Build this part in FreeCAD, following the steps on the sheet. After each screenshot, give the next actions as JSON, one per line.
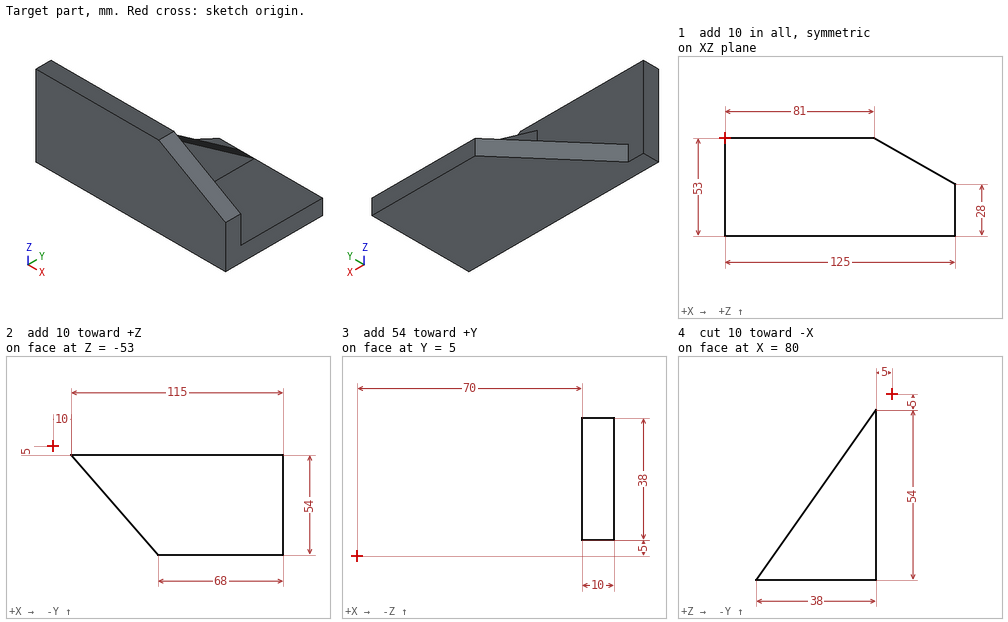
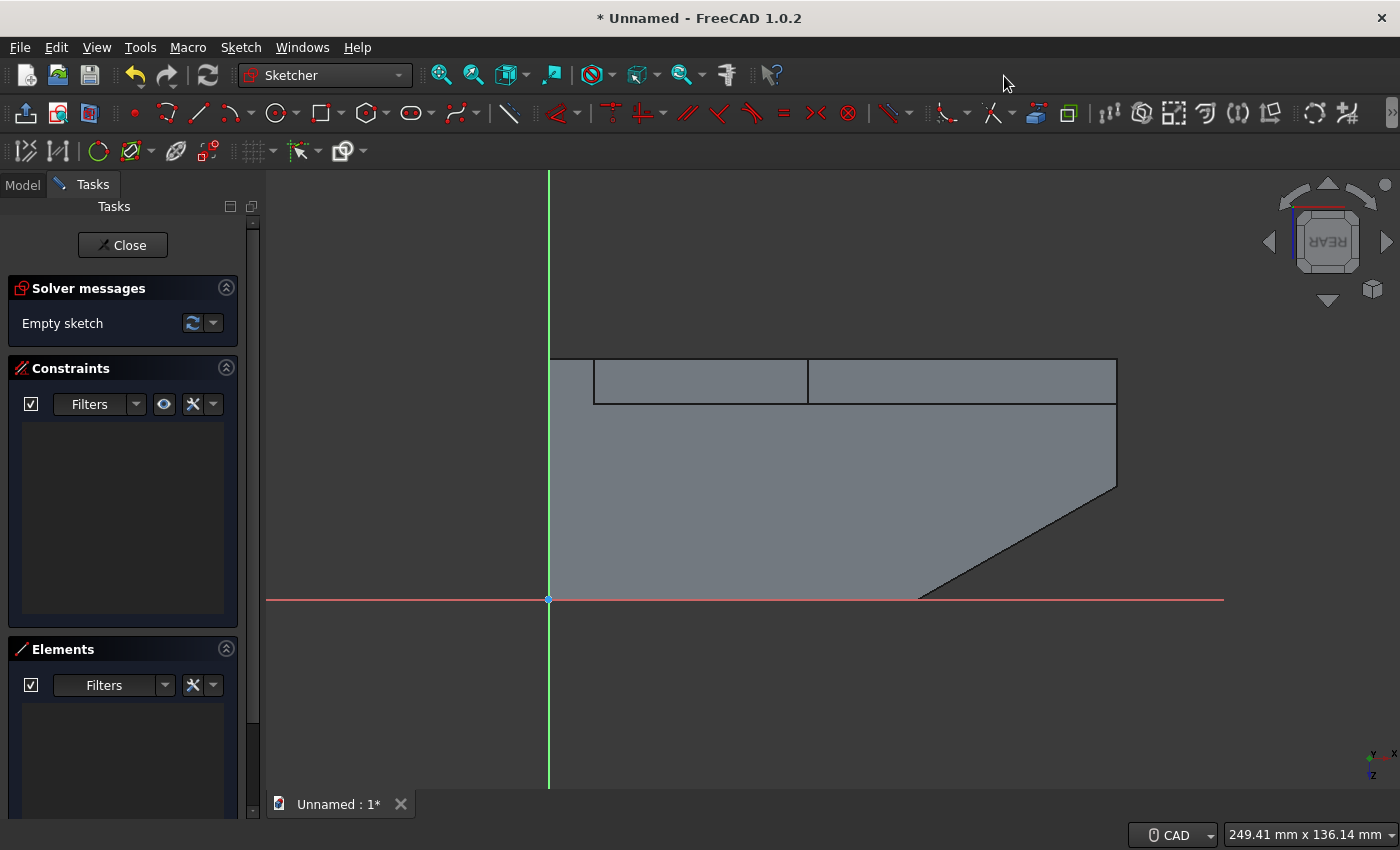
{"action": "scroll", "coordinate": [690, 530], "scroll_direction": "up", "scroll_amount": 3}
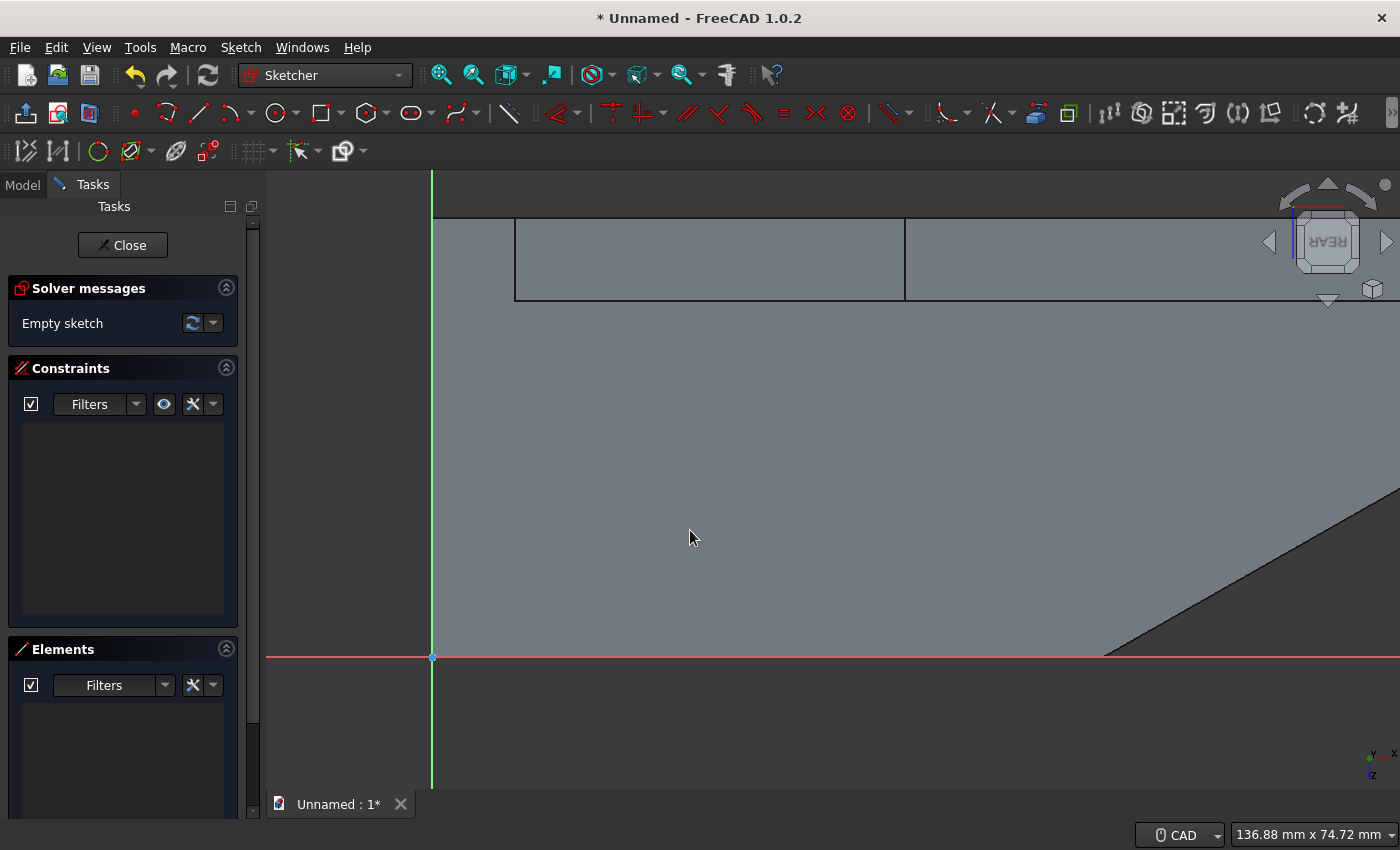
{"action": "left_click", "coordinate": [322, 114]}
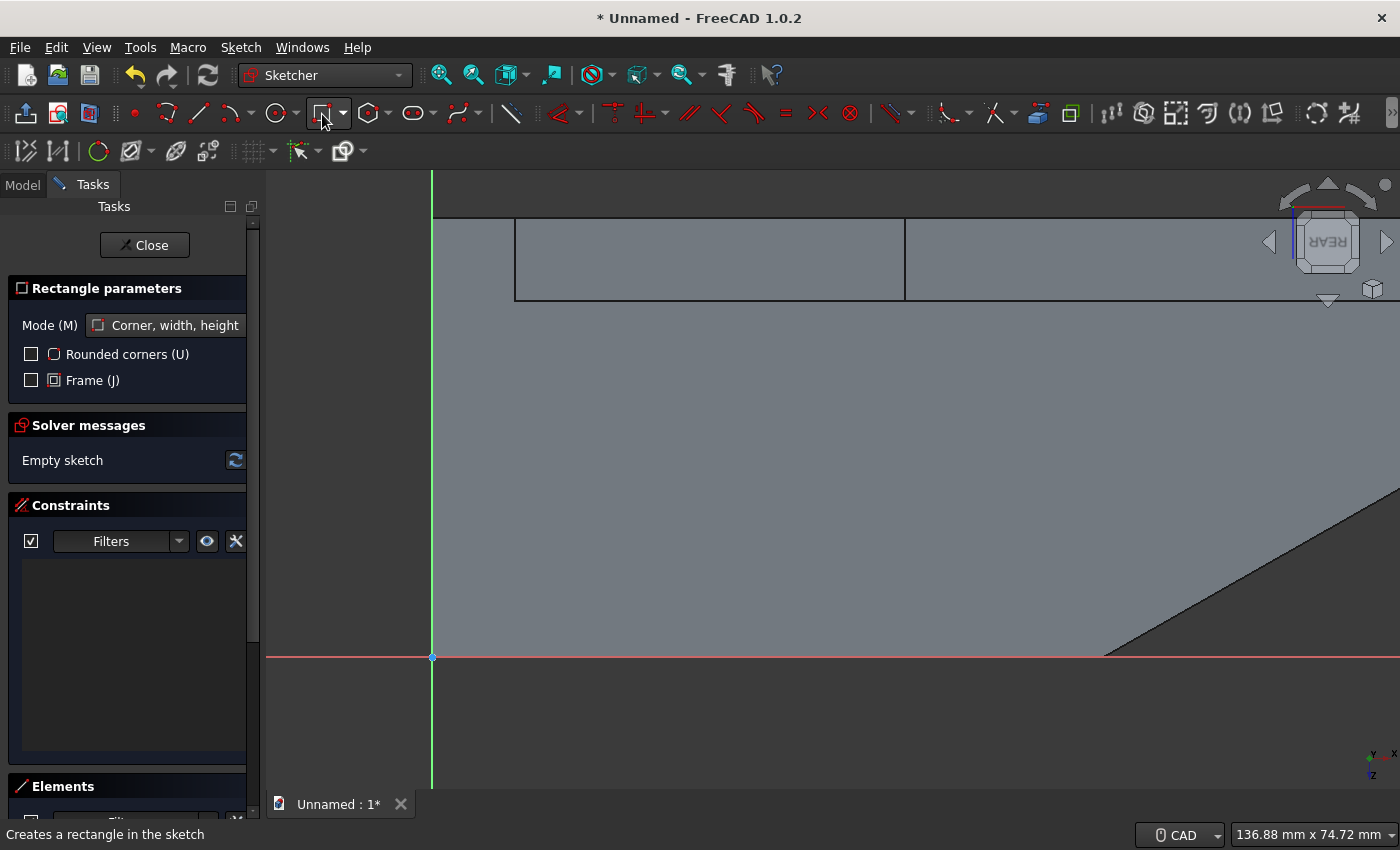
{"action": "left_click", "coordinate": [1012, 301]}
{"action": "mouse_move", "coordinate": [1095, 616]}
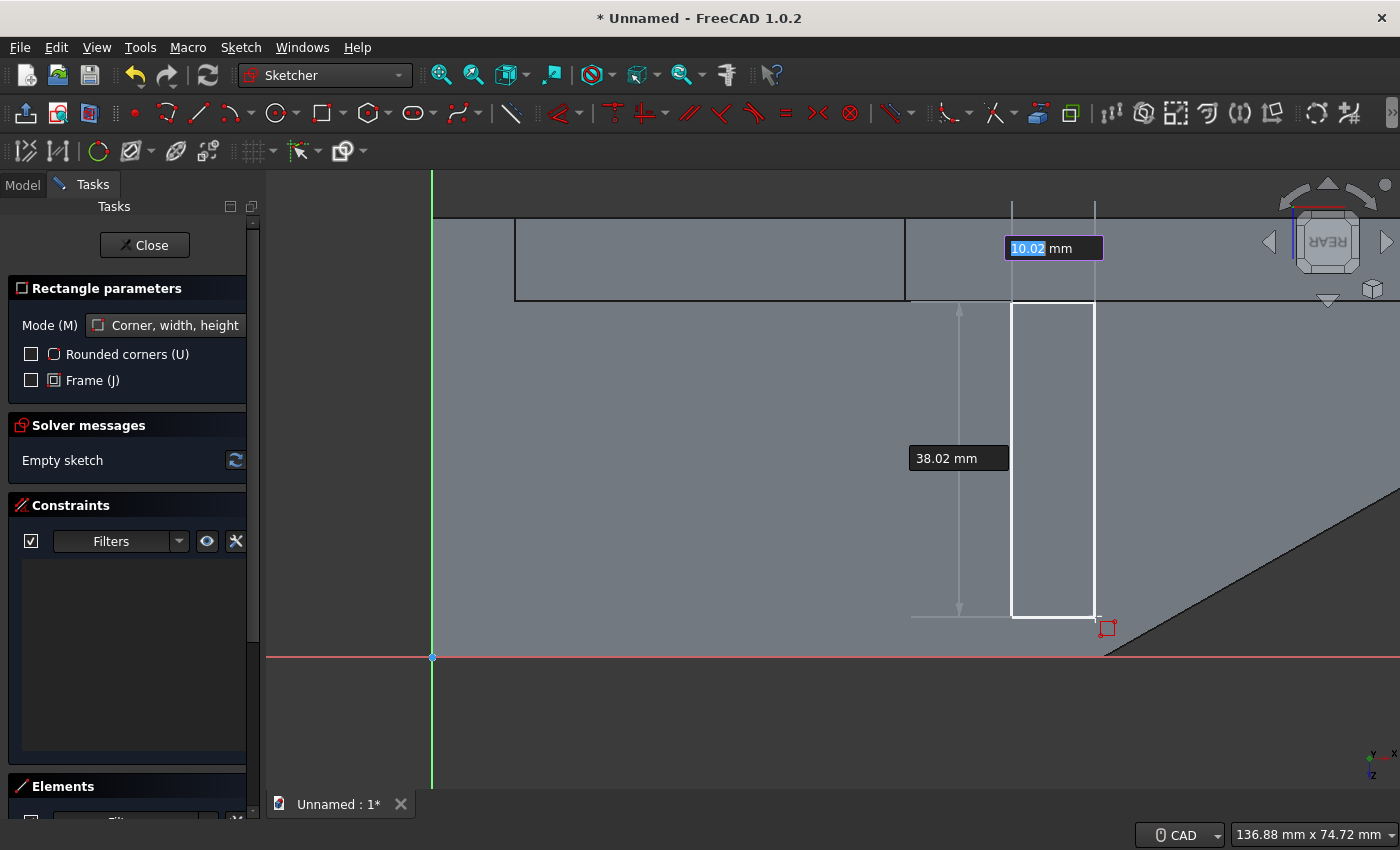
{"action": "type", "text": "10"}
{"action": "key", "text": "Tab"}
{"action": "type", "text": "38"}
{"action": "key", "text": "Return"}
{"action": "key", "text": "Escape"}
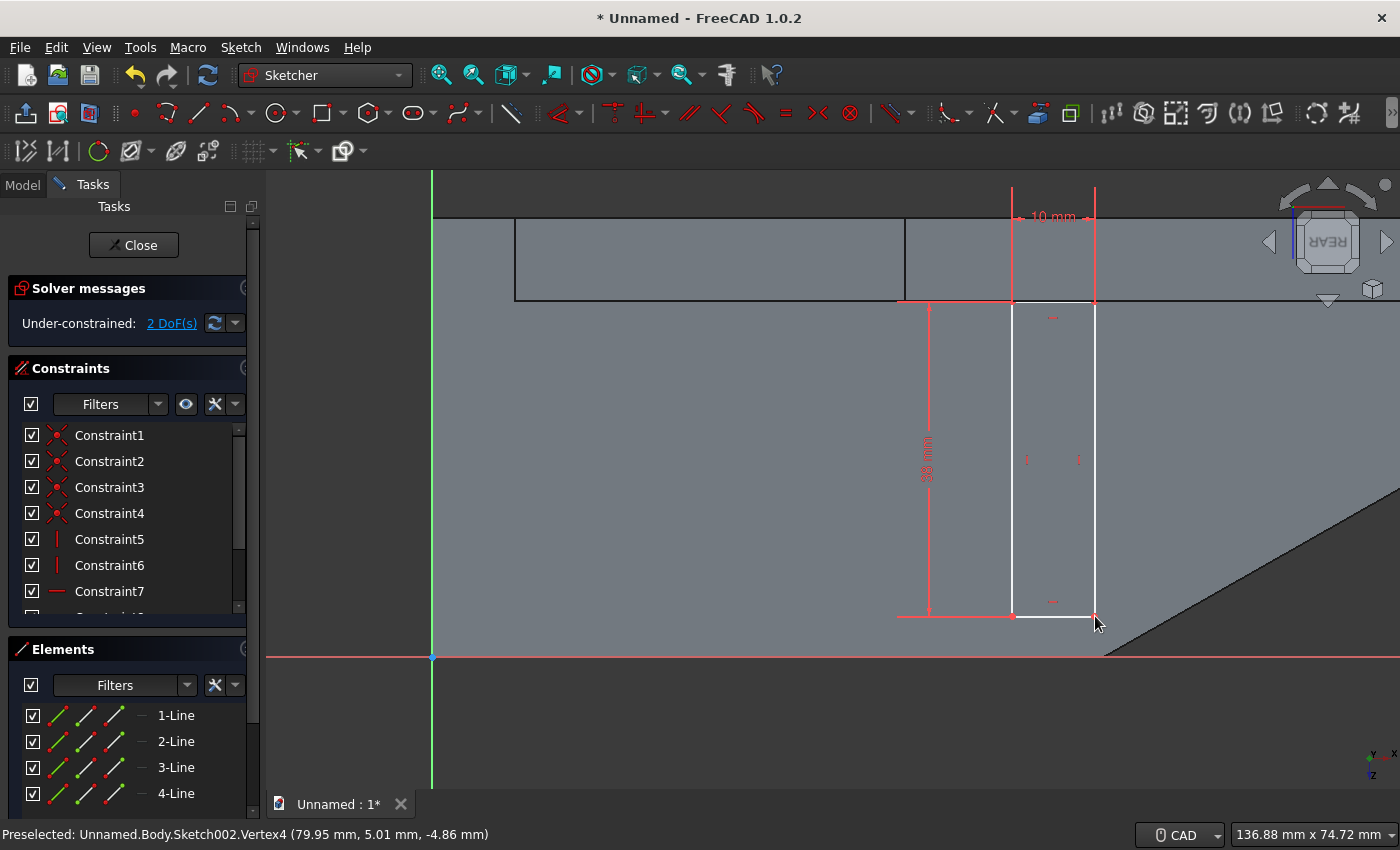
{"action": "key", "text": "d"}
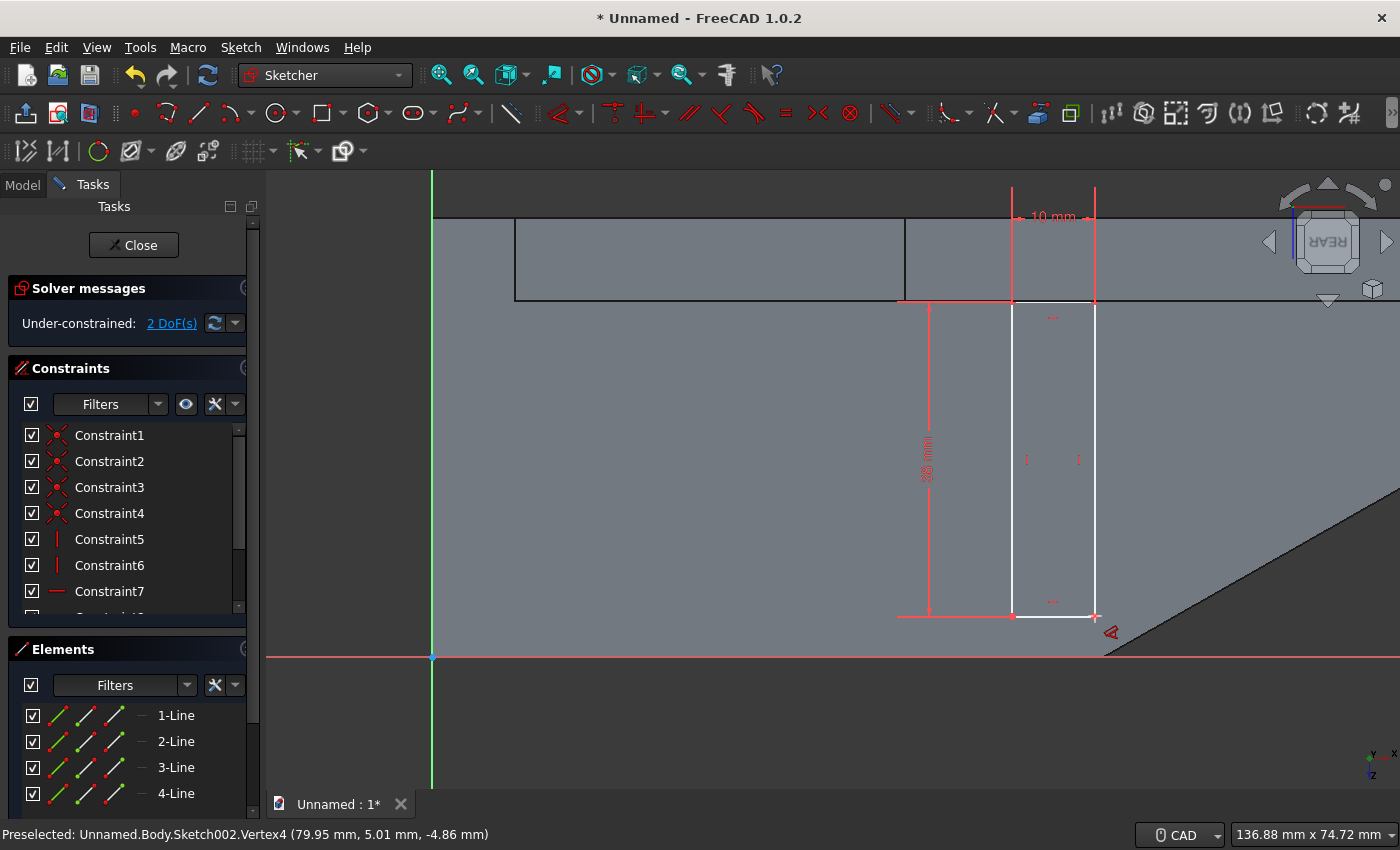
{"action": "left_click", "coordinate": [1012, 617]}
{"action": "left_click", "coordinate": [398, 637]}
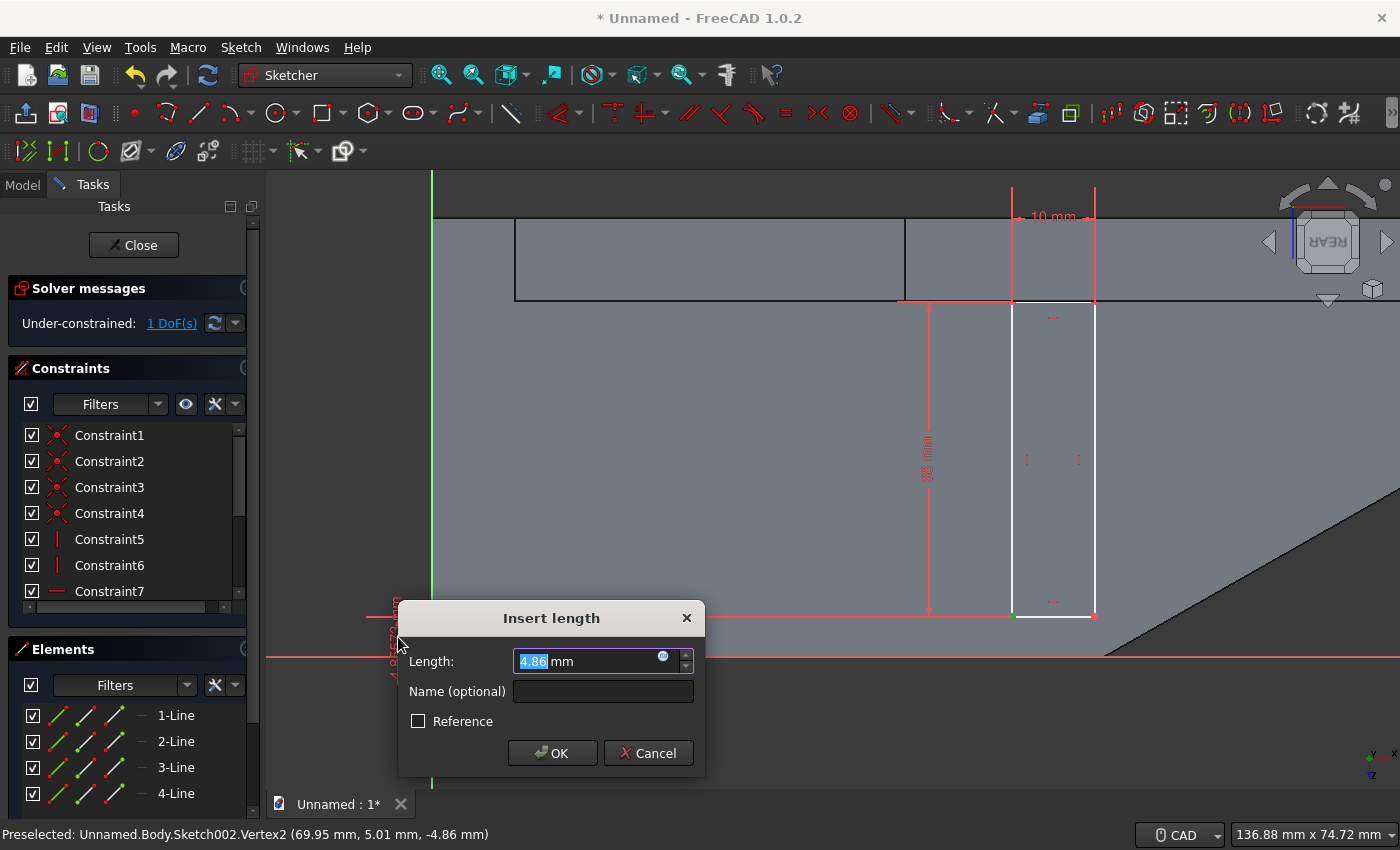
{"action": "type", "text": "5"}
{"action": "key", "text": "Return"}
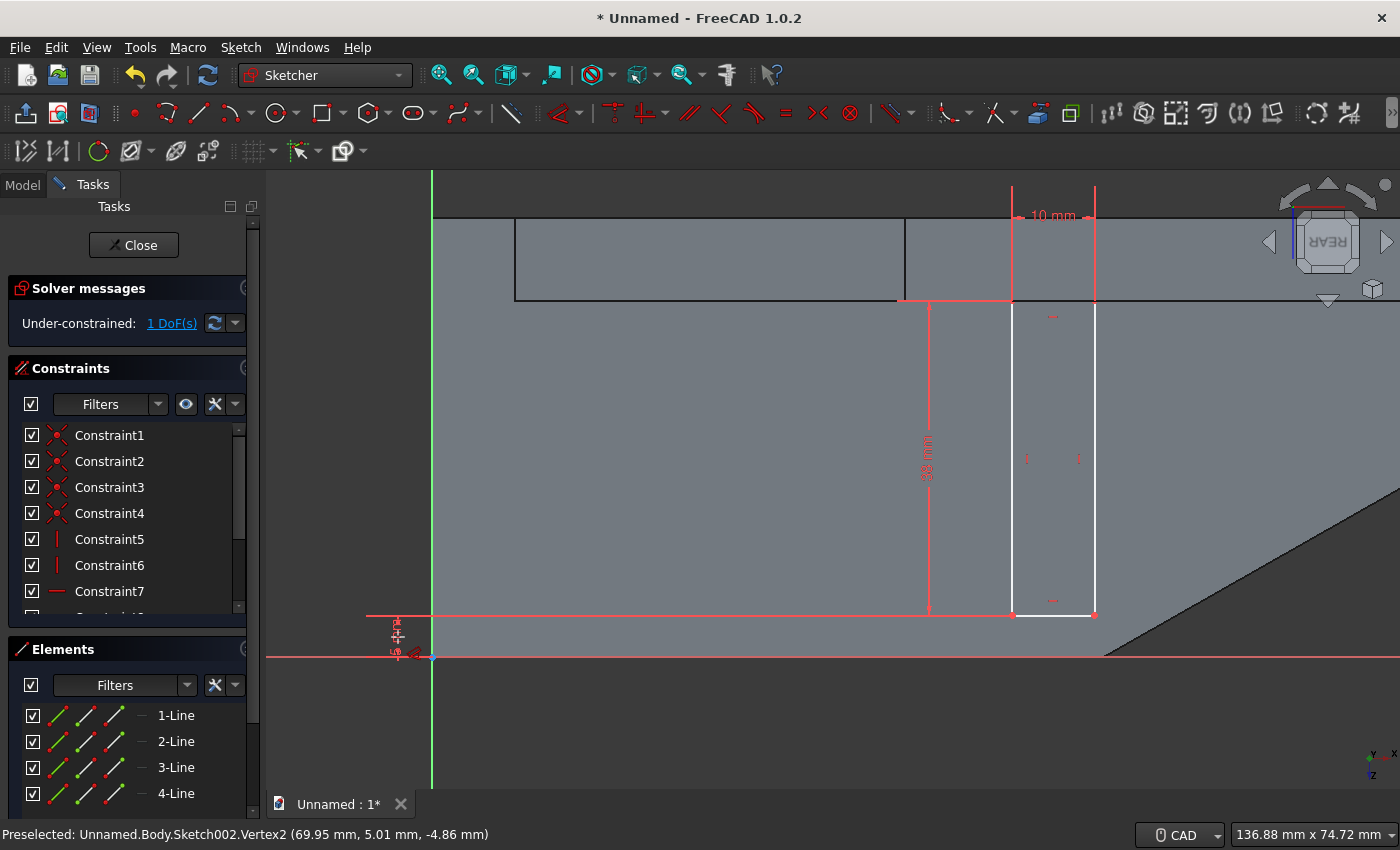
{"action": "left_click", "coordinate": [1012, 301]}
{"action": "left_click", "coordinate": [722, 691]}